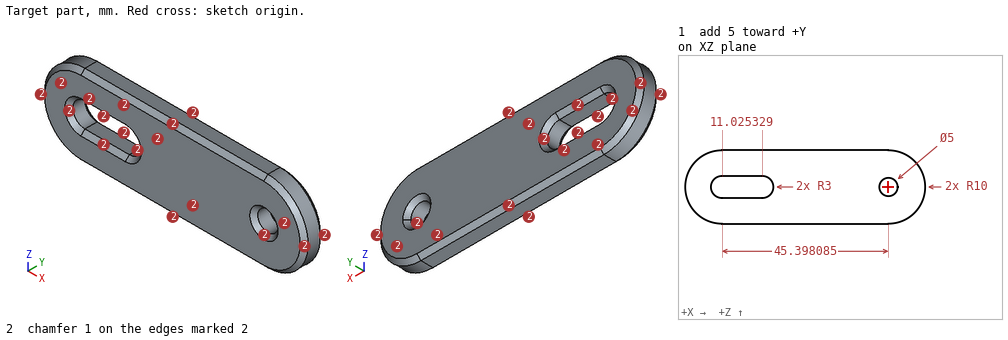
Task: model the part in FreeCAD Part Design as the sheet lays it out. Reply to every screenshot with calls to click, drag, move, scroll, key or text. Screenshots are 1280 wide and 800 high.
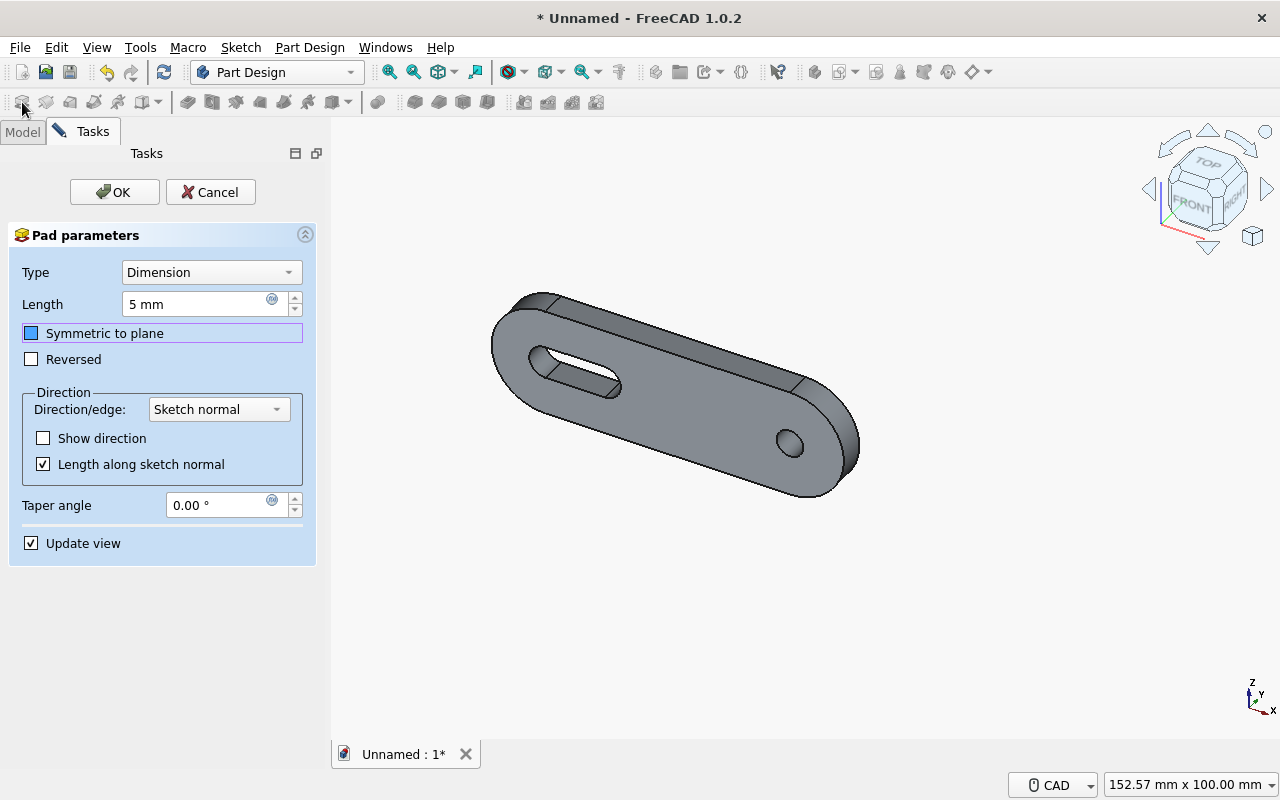
click(30, 359)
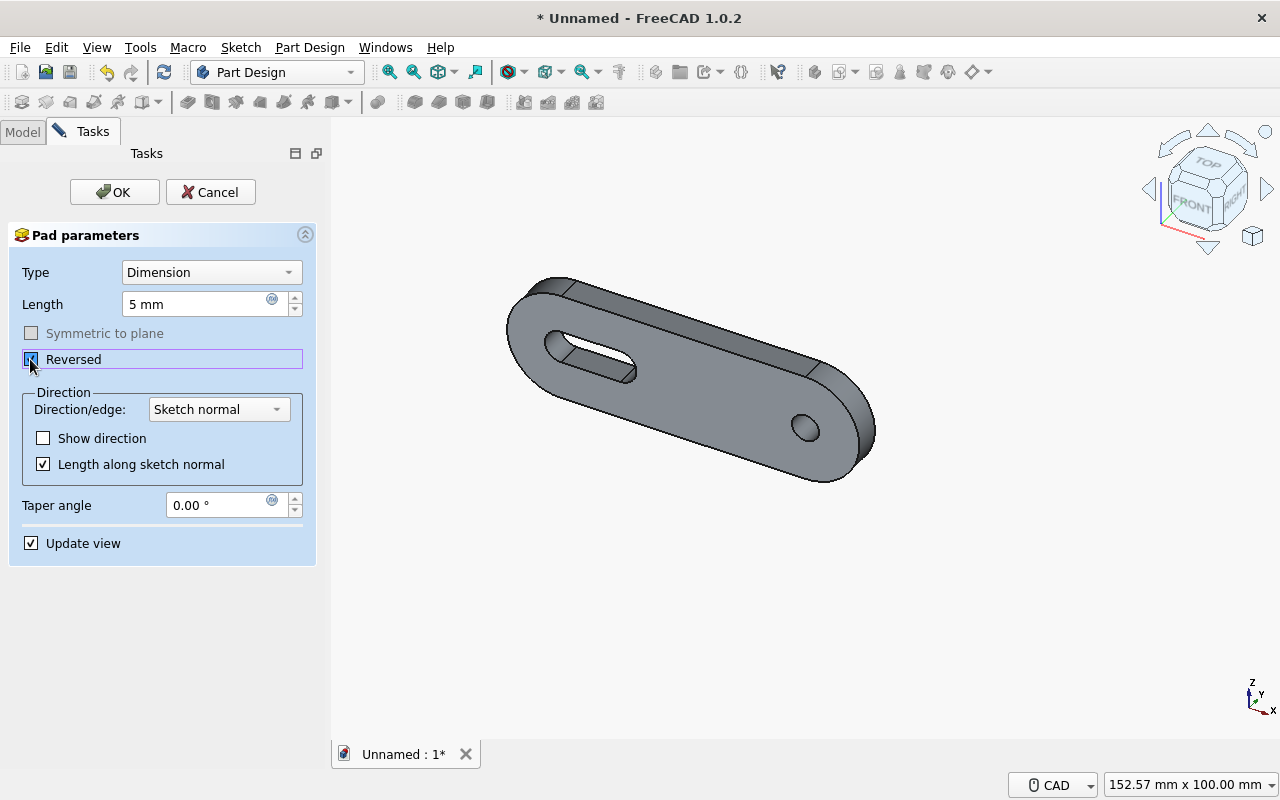
click(115, 192)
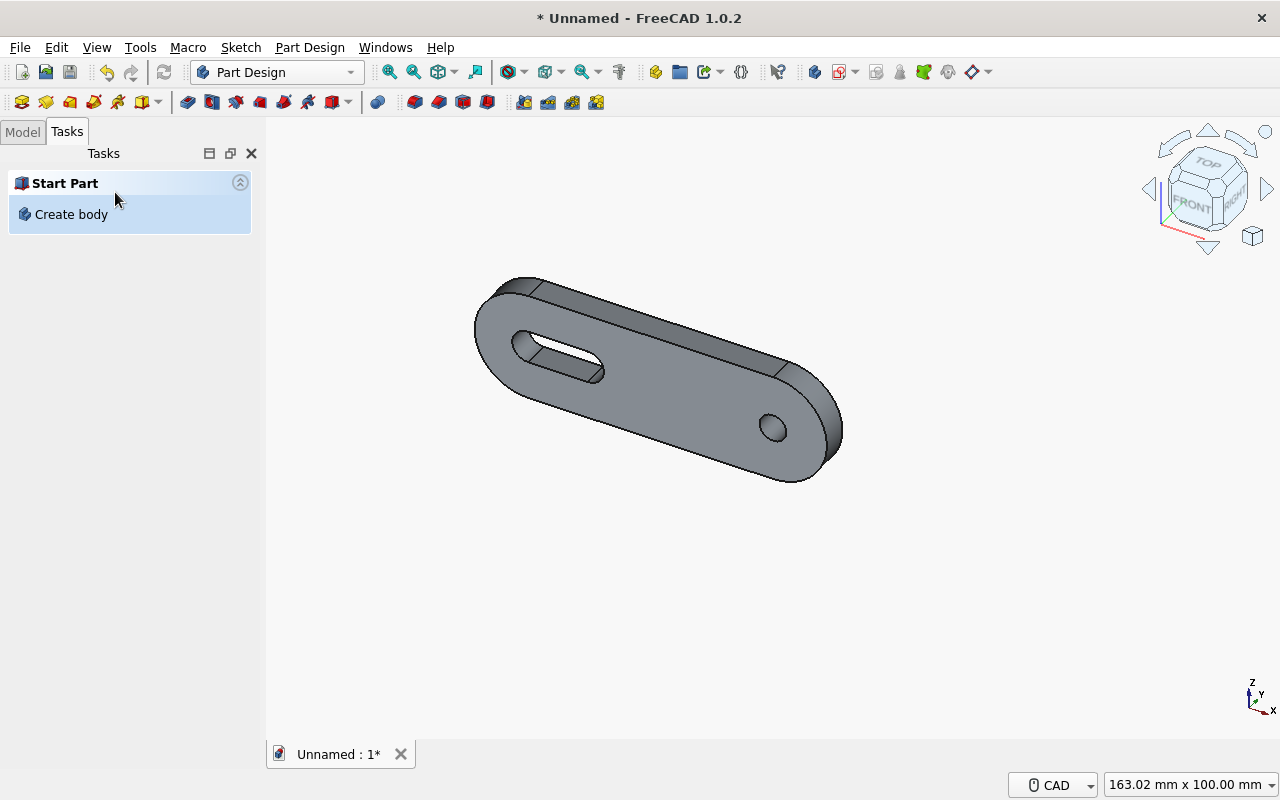
click(390, 72)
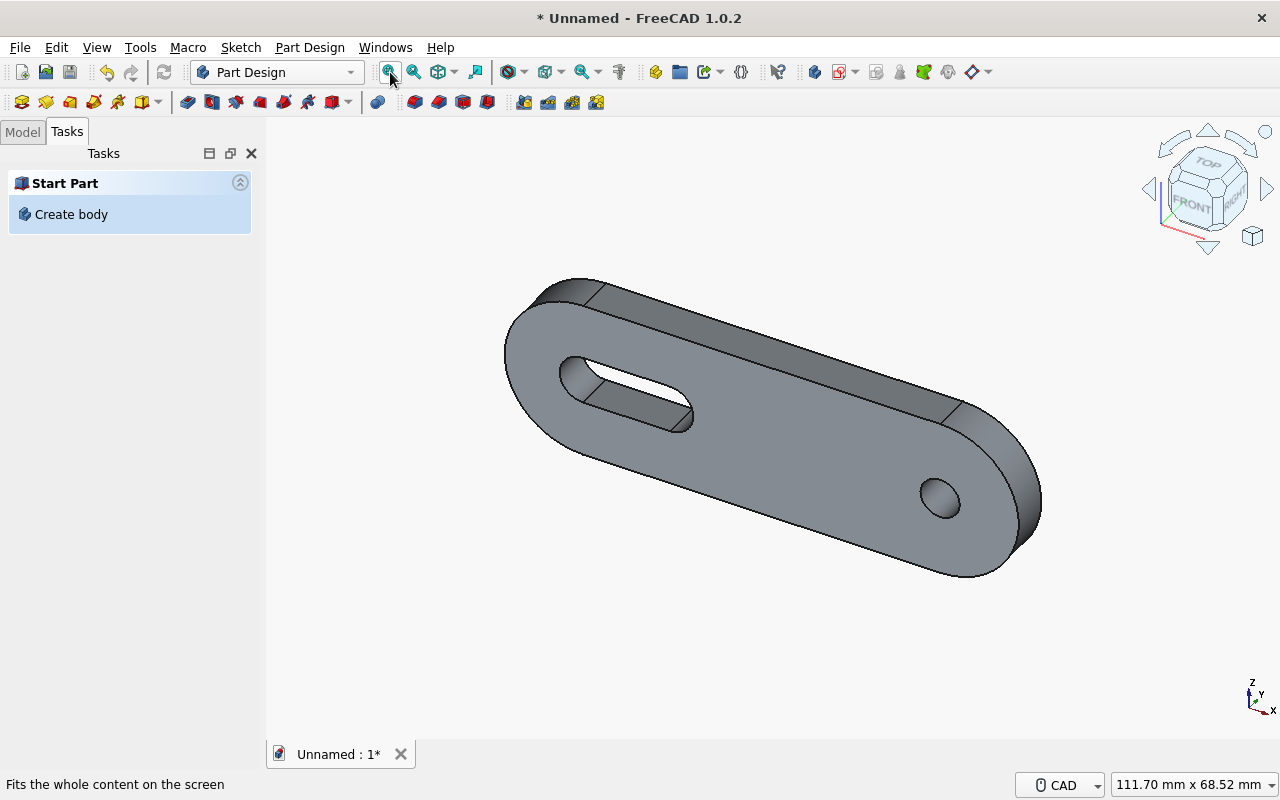
click(835, 463)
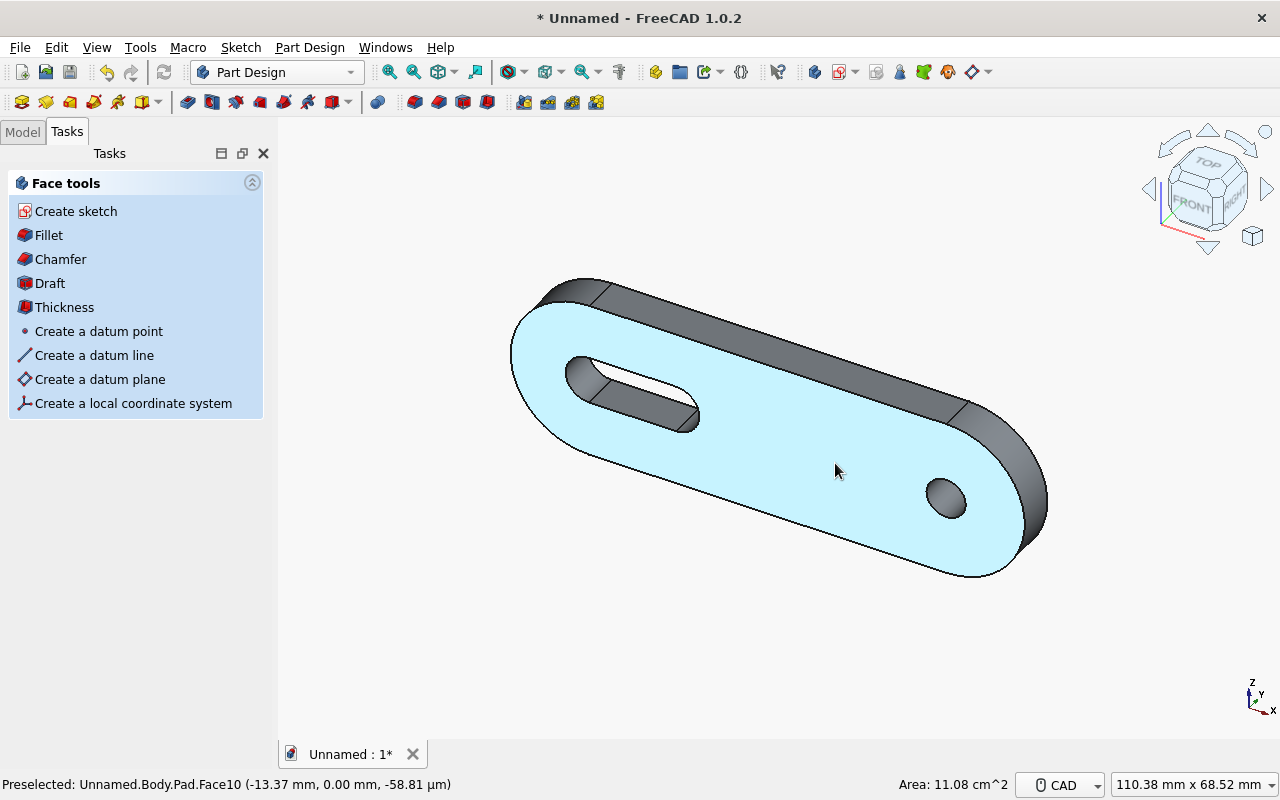
key(0)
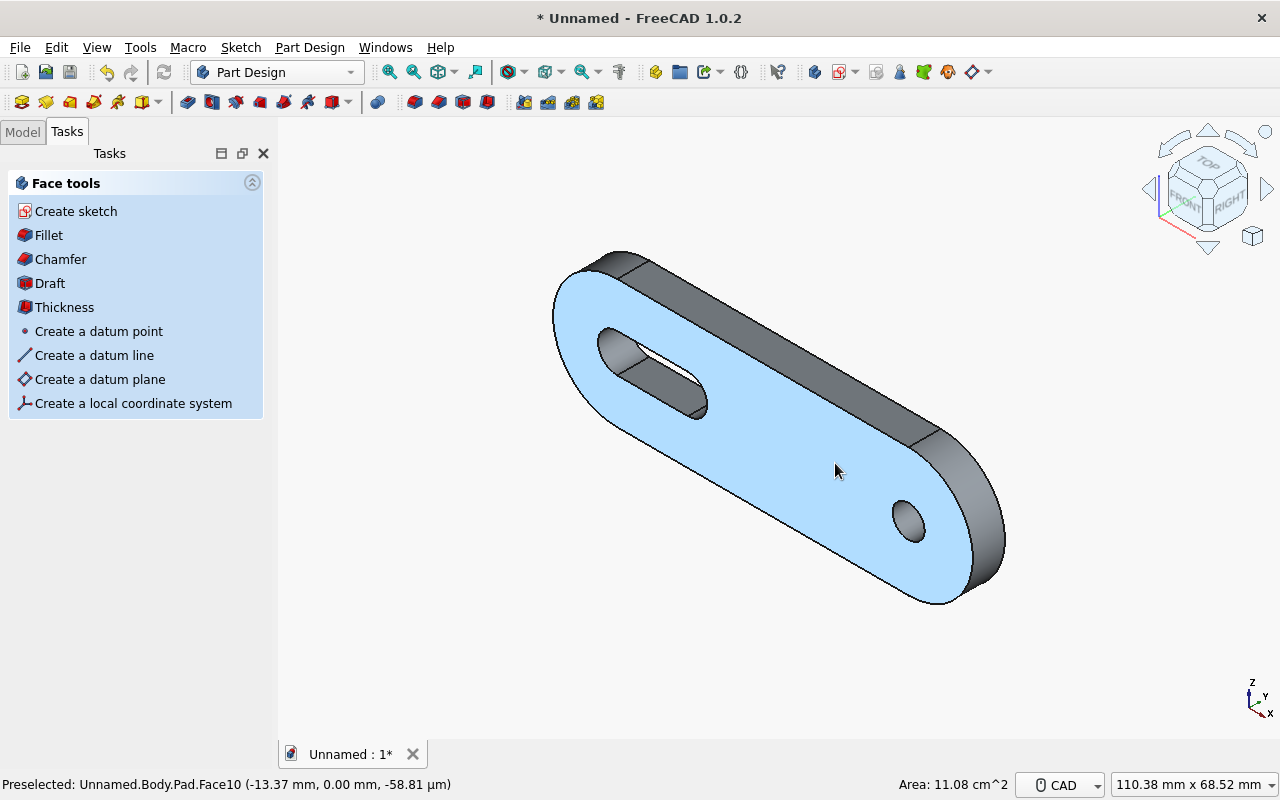
key(2)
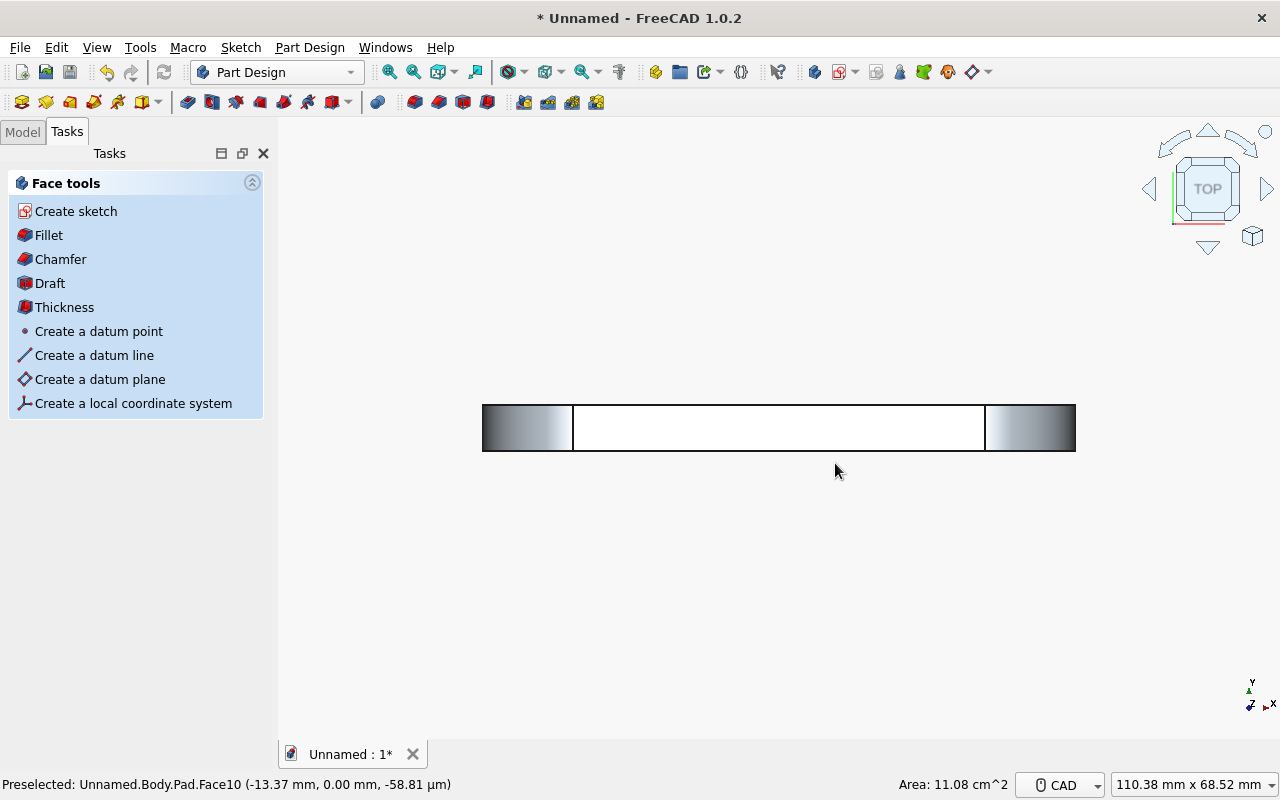
key(1)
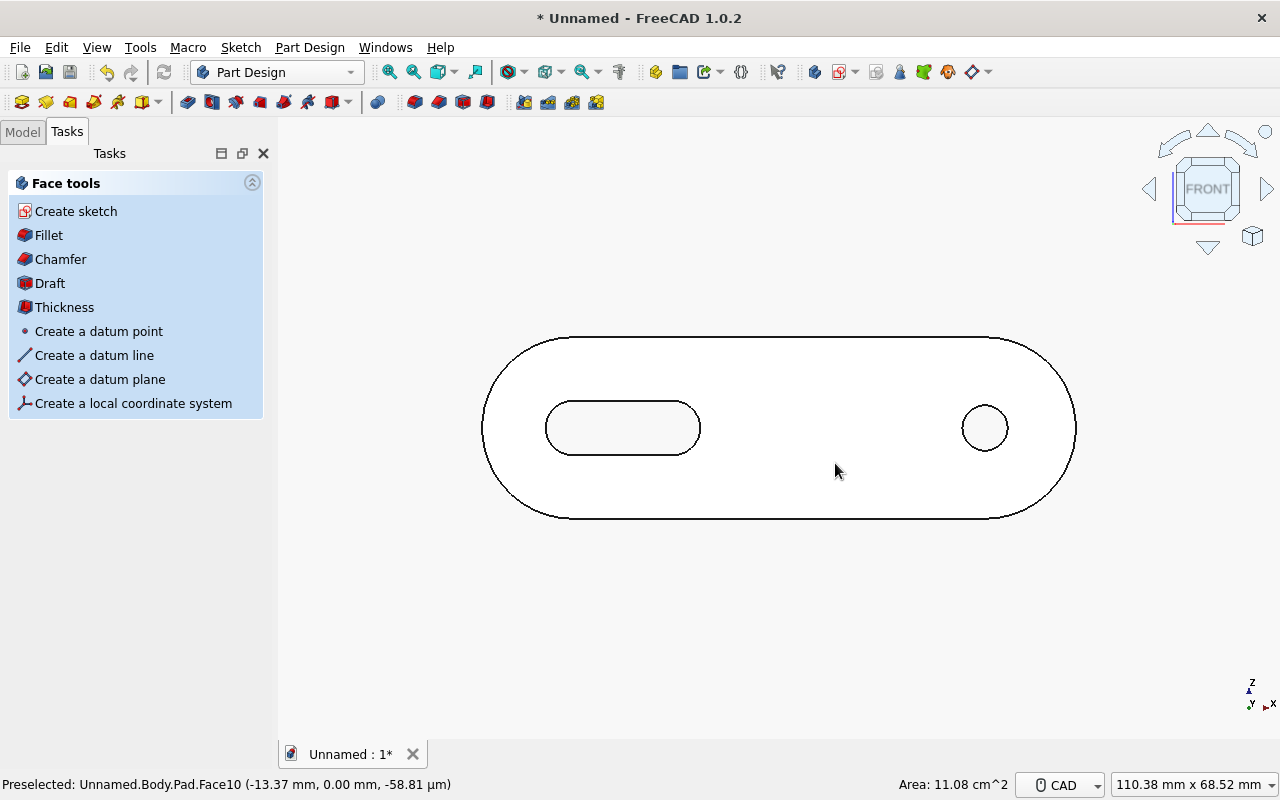
key(3)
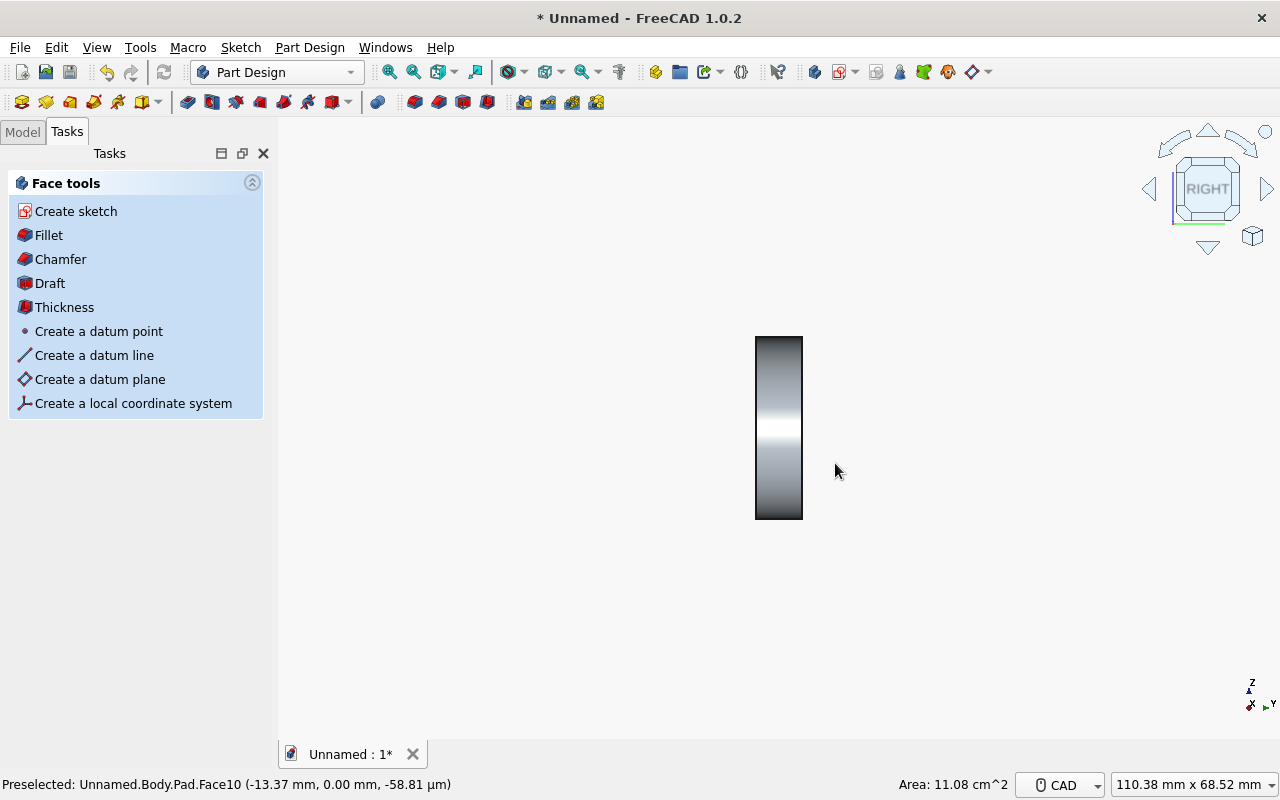
click(390, 72)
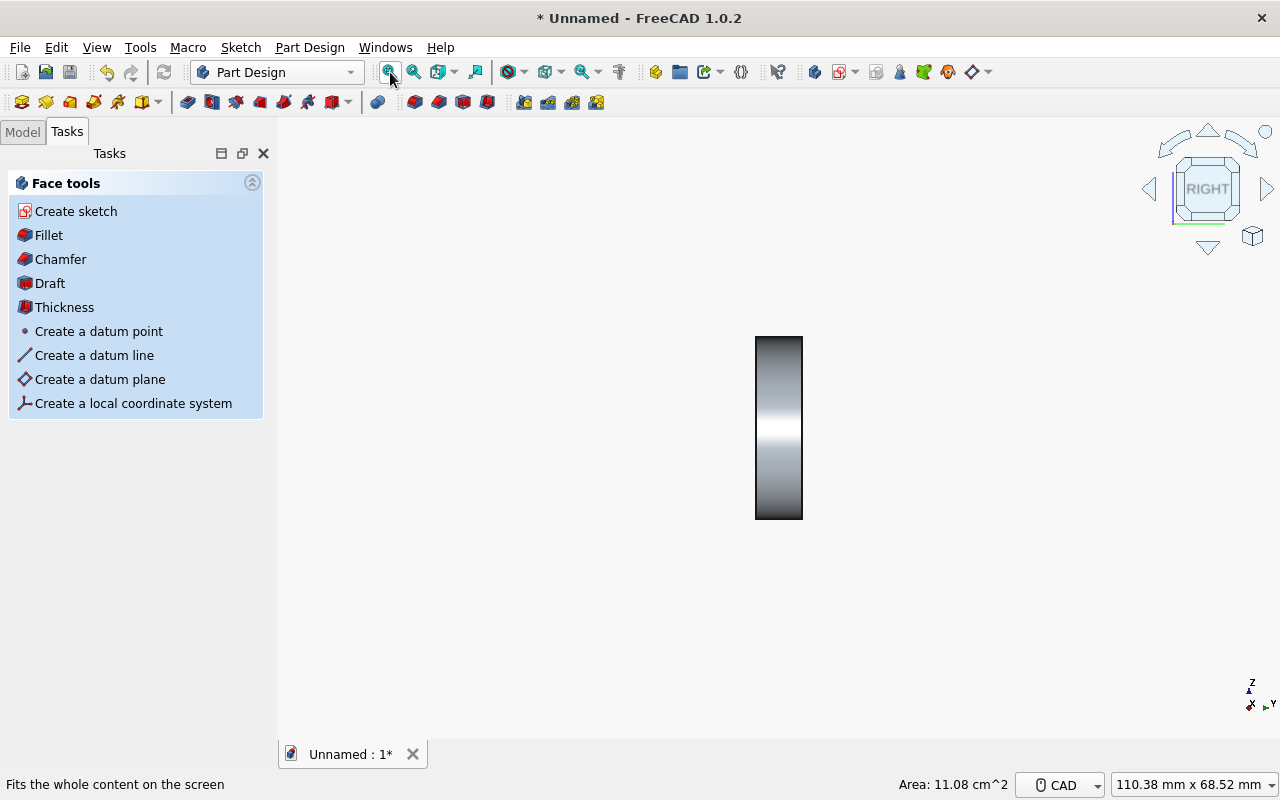
key(5)